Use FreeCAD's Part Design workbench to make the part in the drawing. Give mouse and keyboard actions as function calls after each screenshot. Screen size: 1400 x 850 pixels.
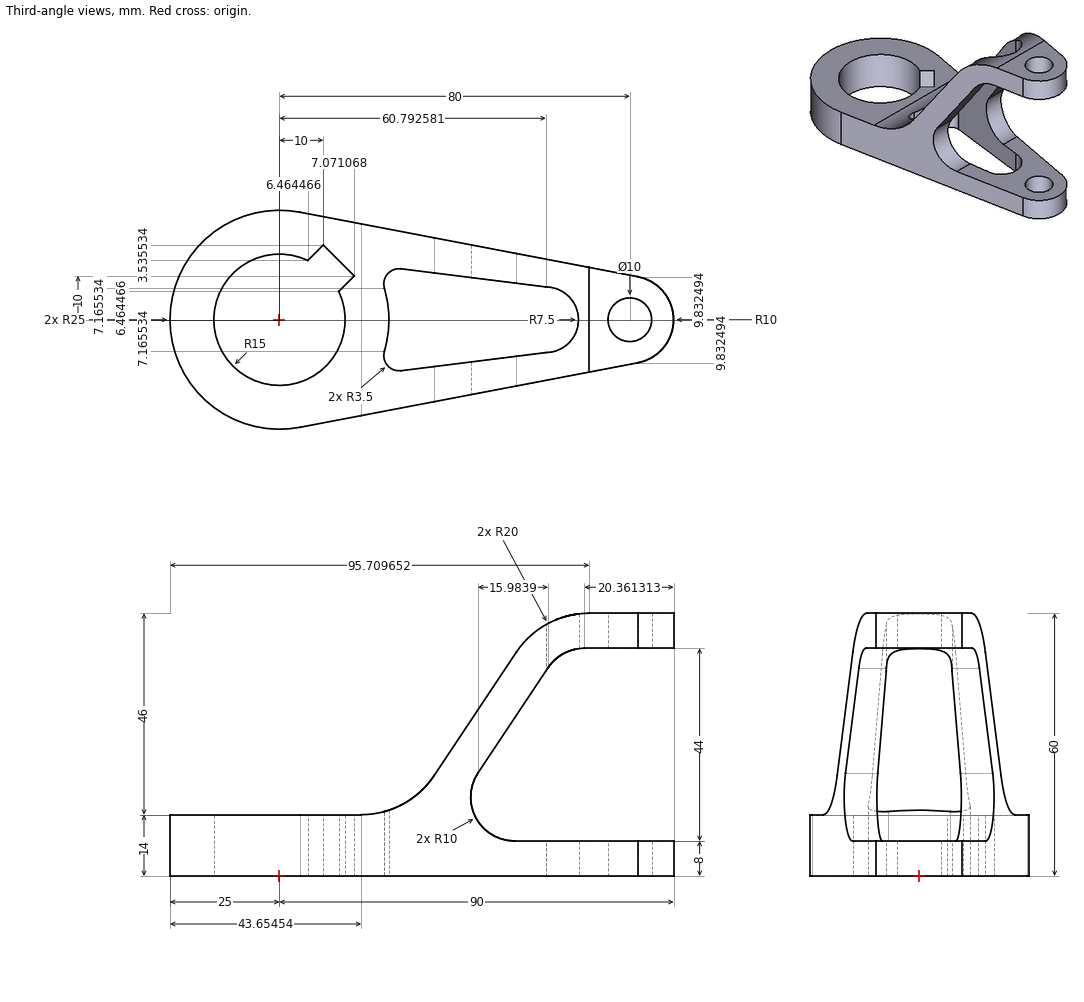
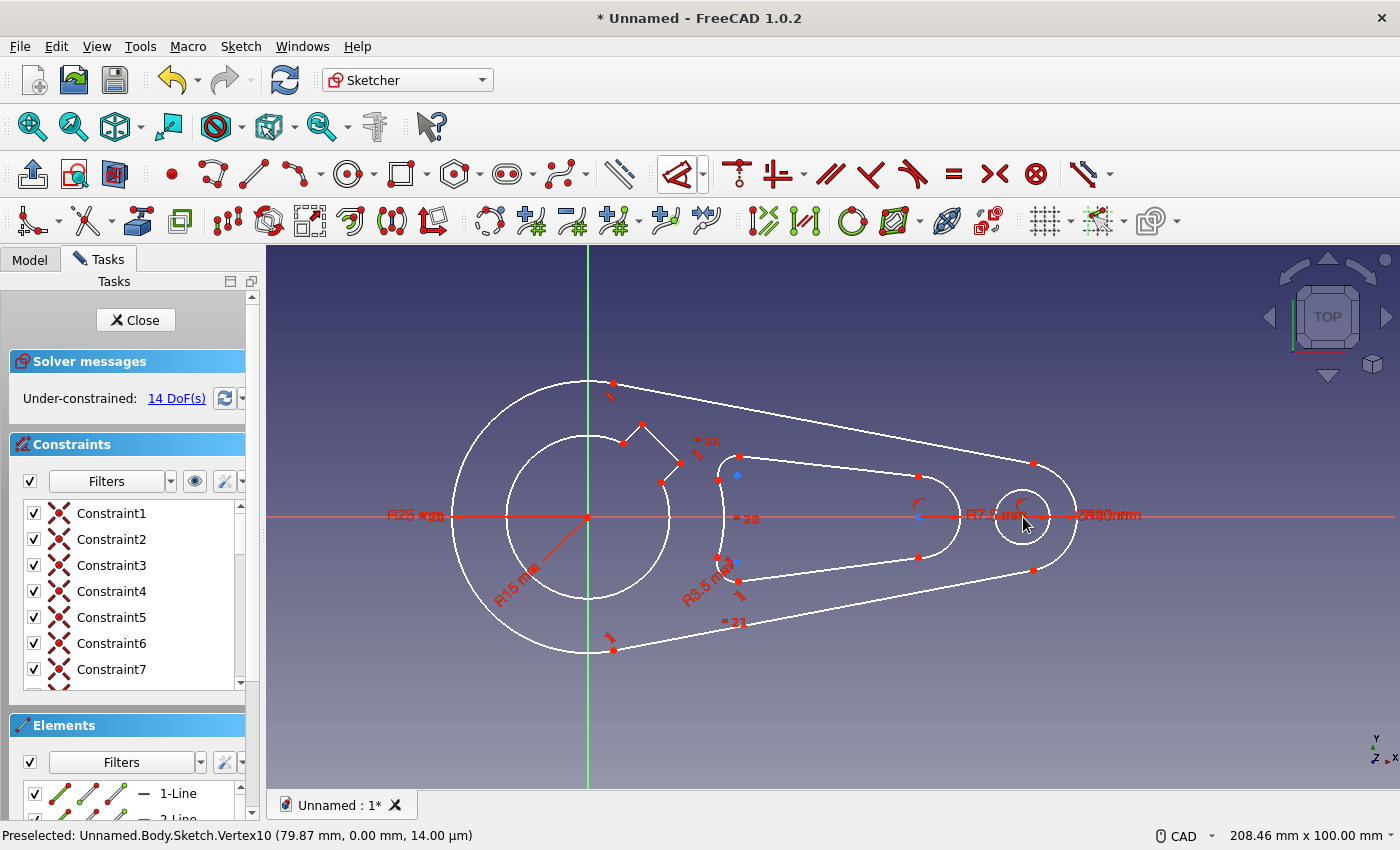
key(l)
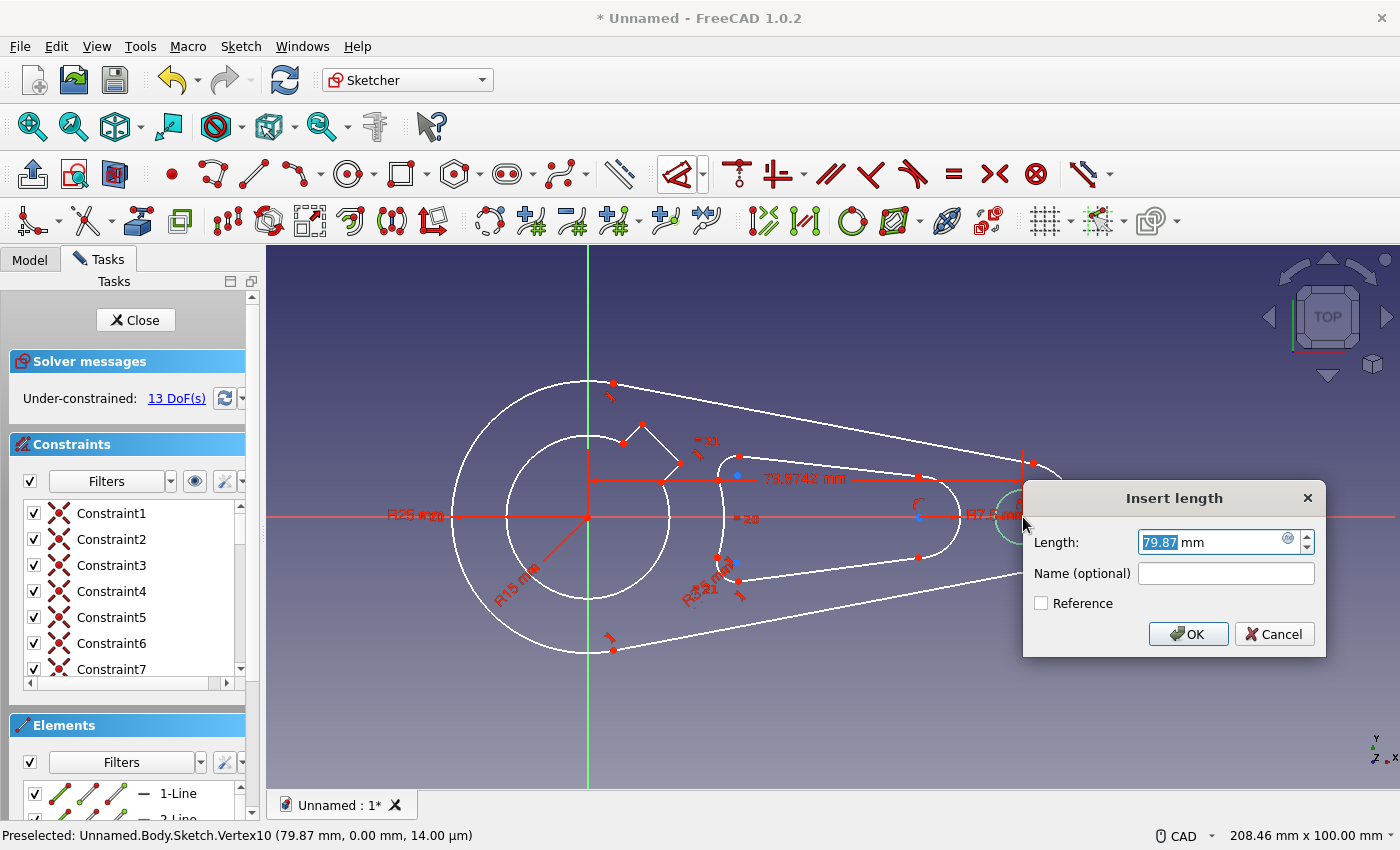
text(80)
key(Return)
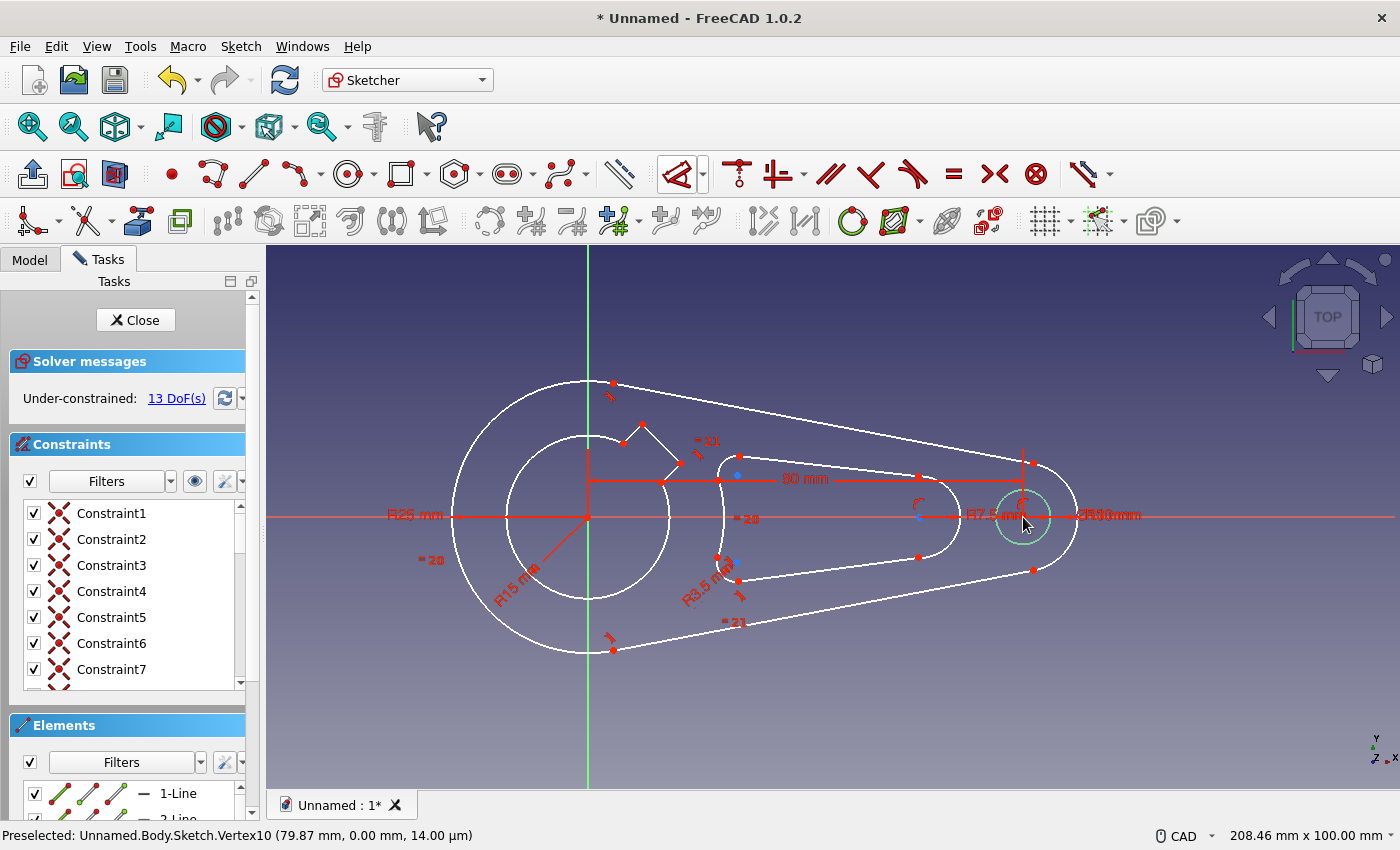
click(642, 425)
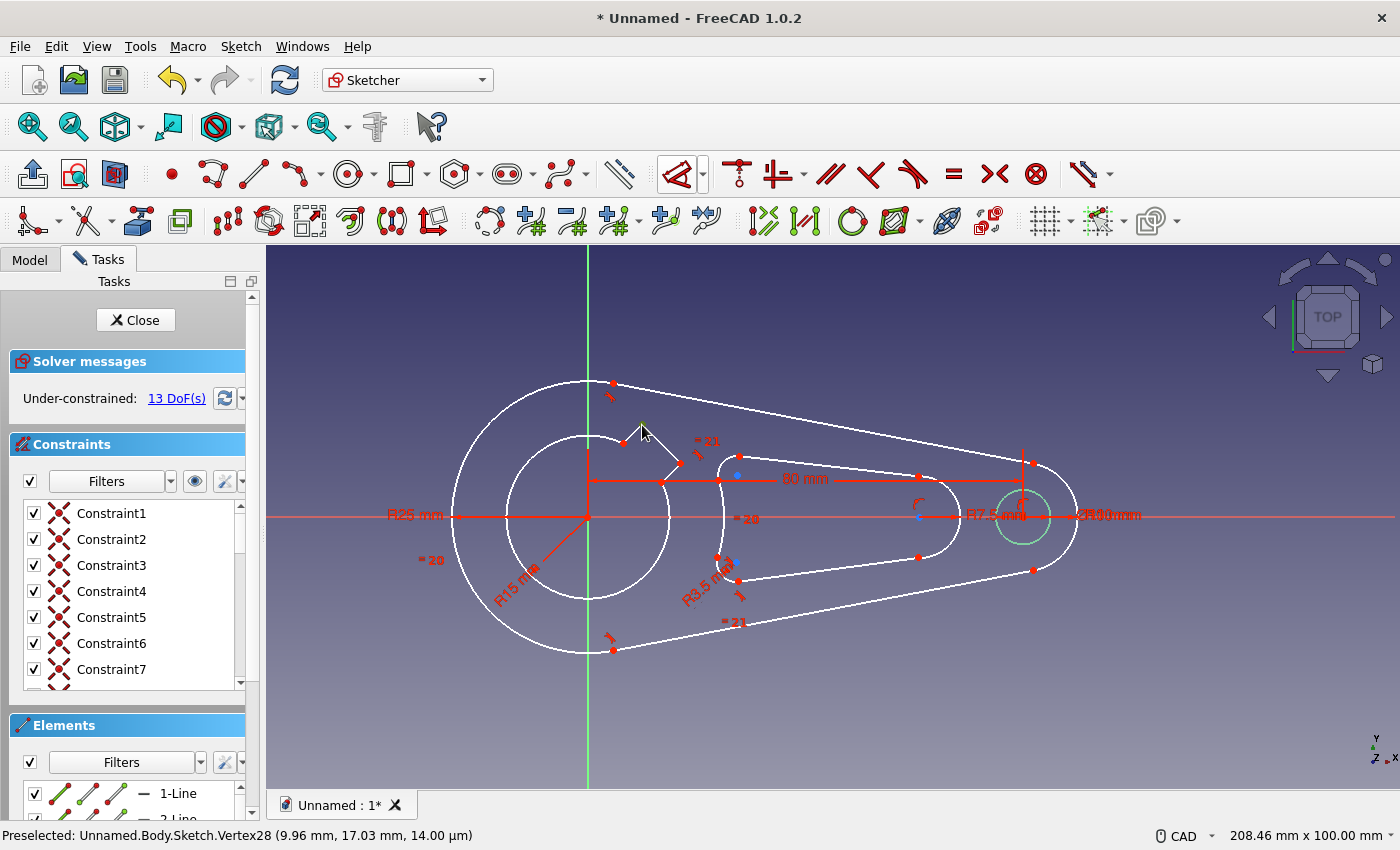
click(702, 174)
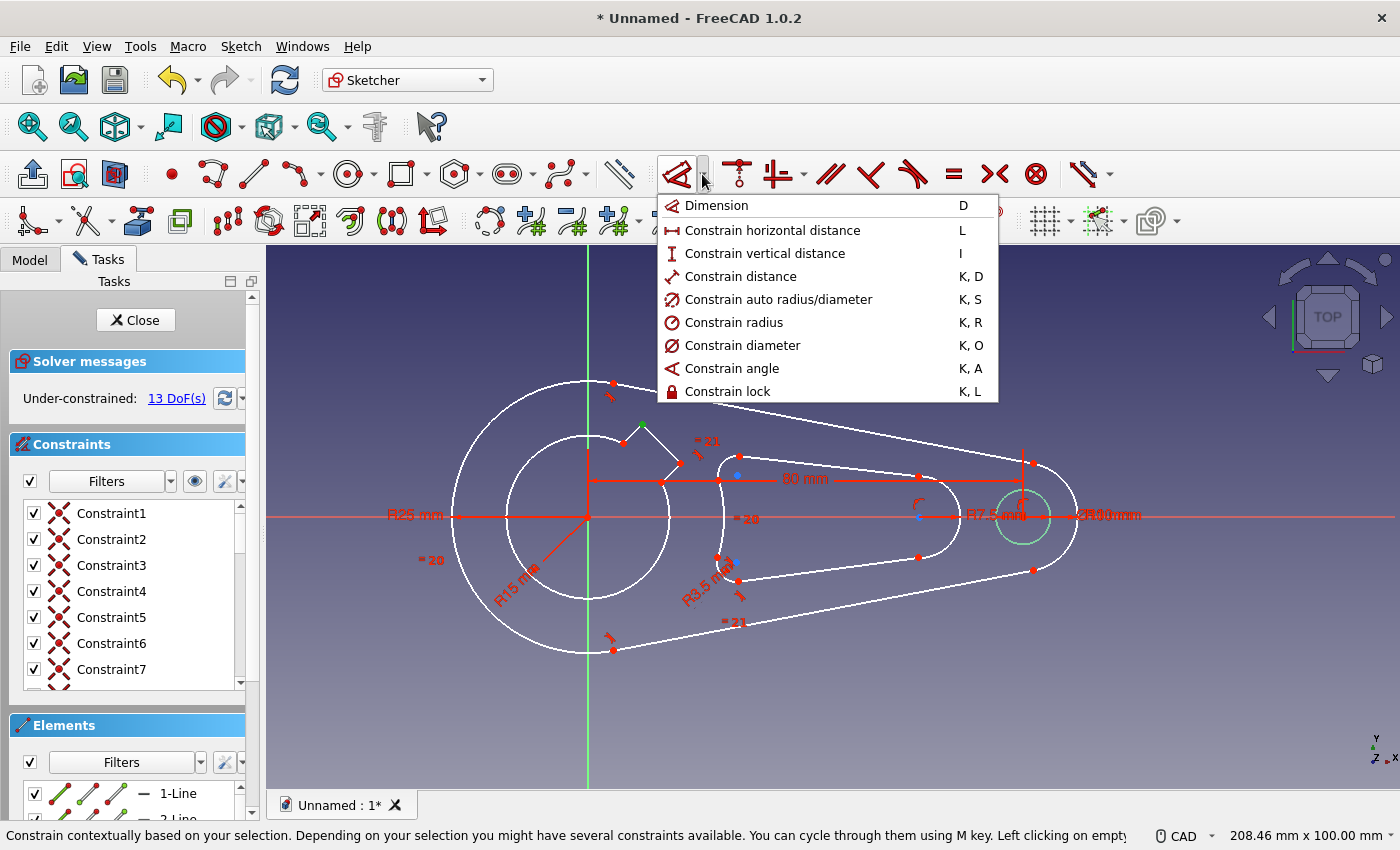
click(828, 230)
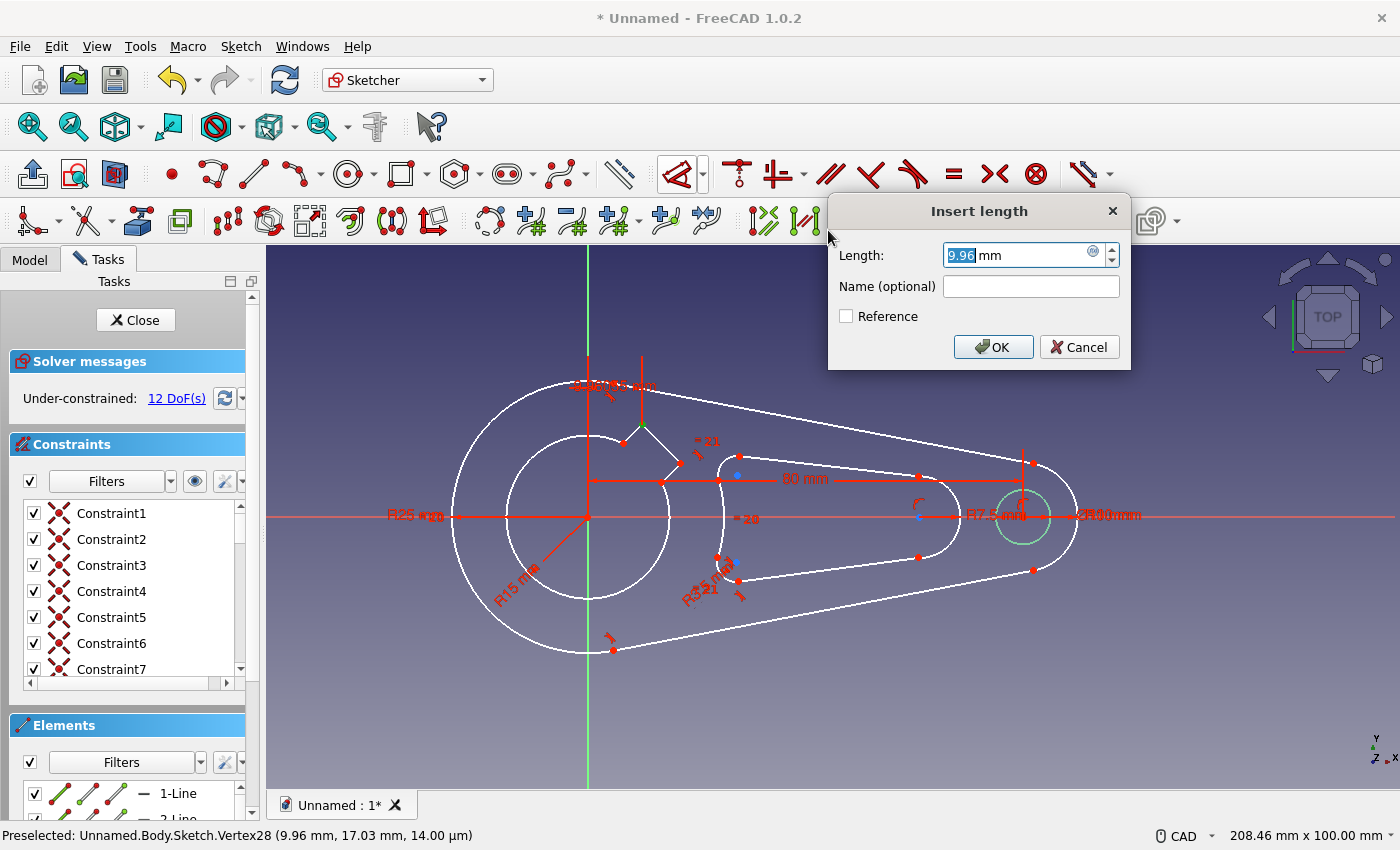
text(10)
key(Return)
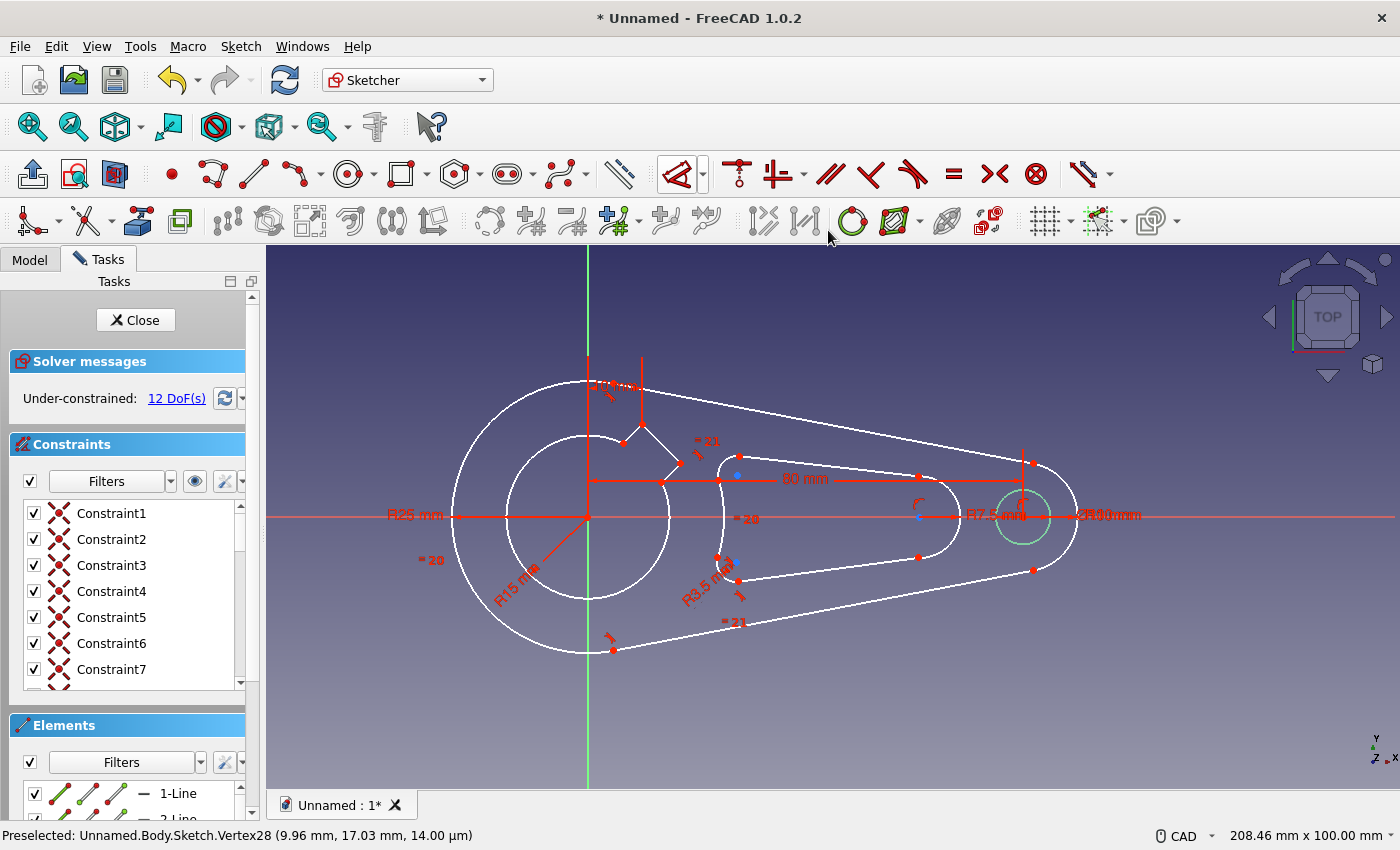
click(681, 463)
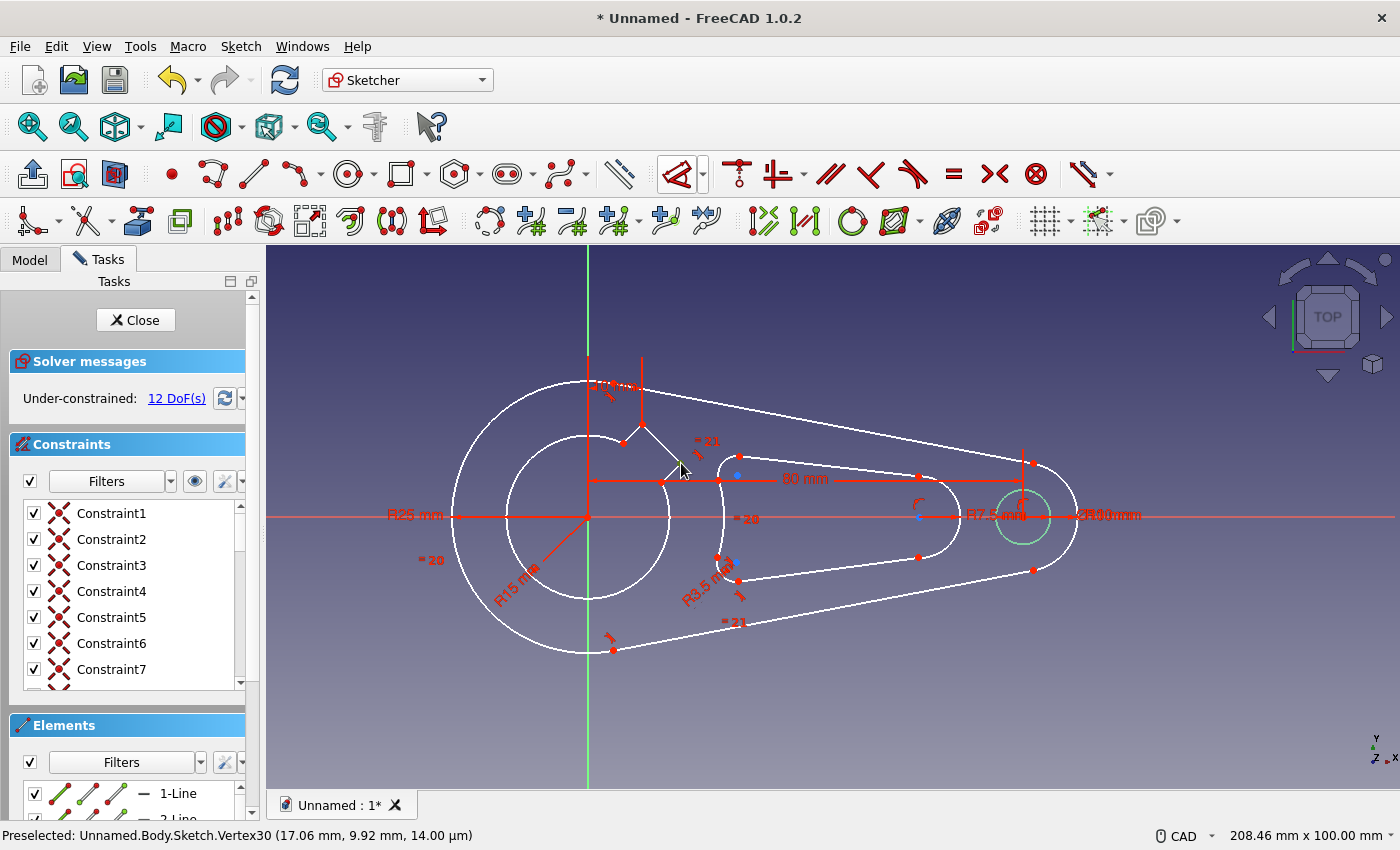
click(702, 174)